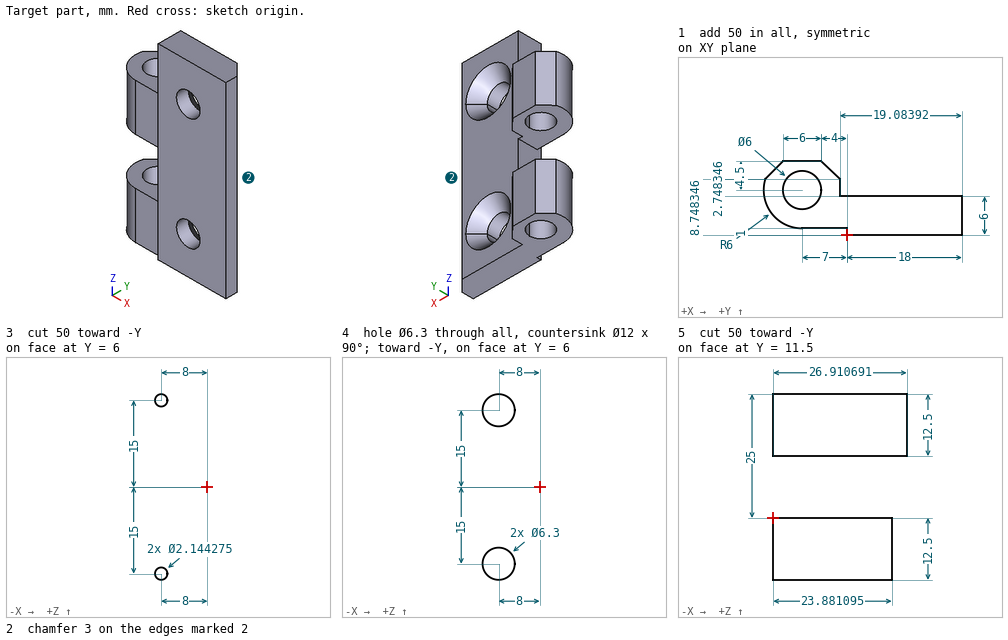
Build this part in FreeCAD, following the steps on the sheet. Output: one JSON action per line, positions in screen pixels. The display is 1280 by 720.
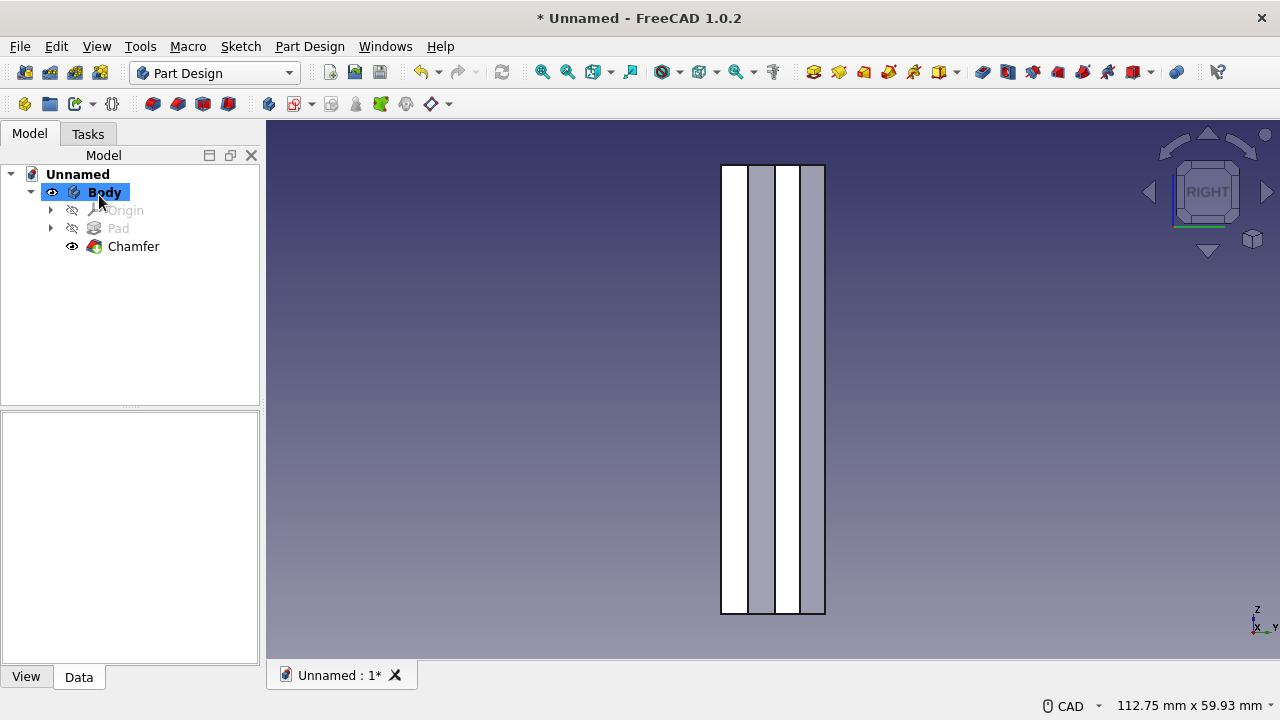
{"action": "key", "text": "4"}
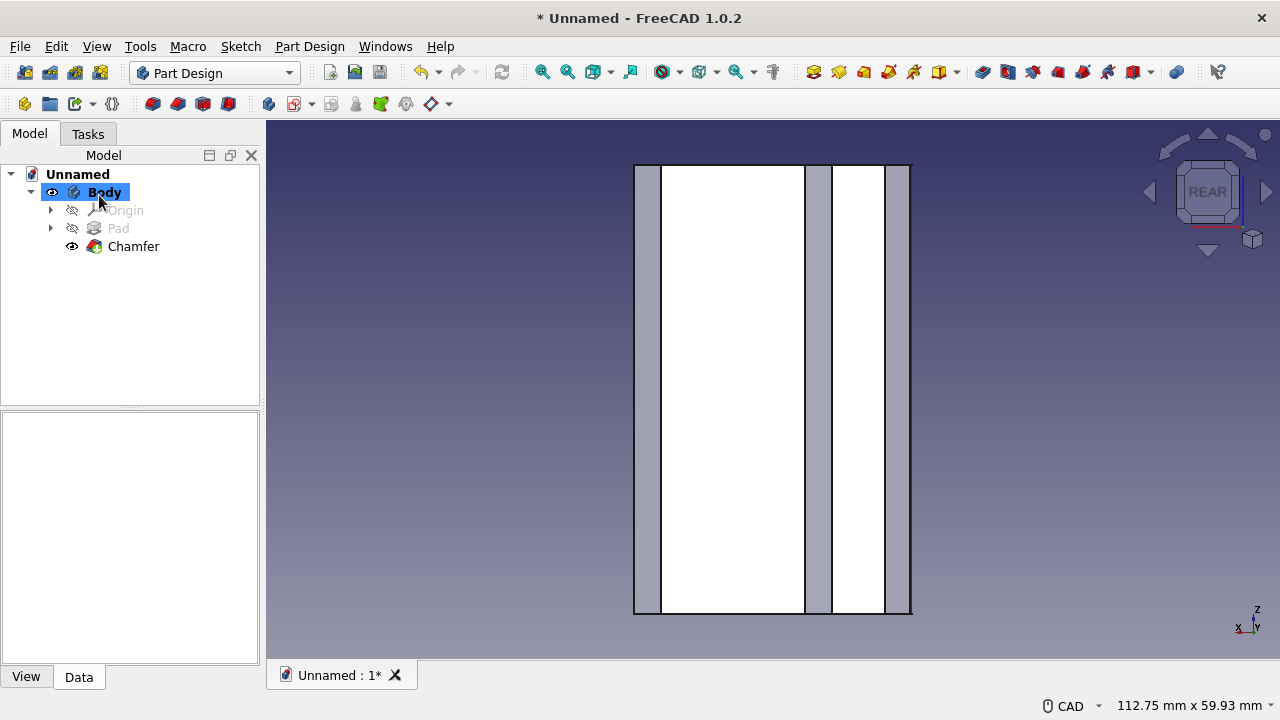
{"action": "left_click", "coordinate": [733, 260]}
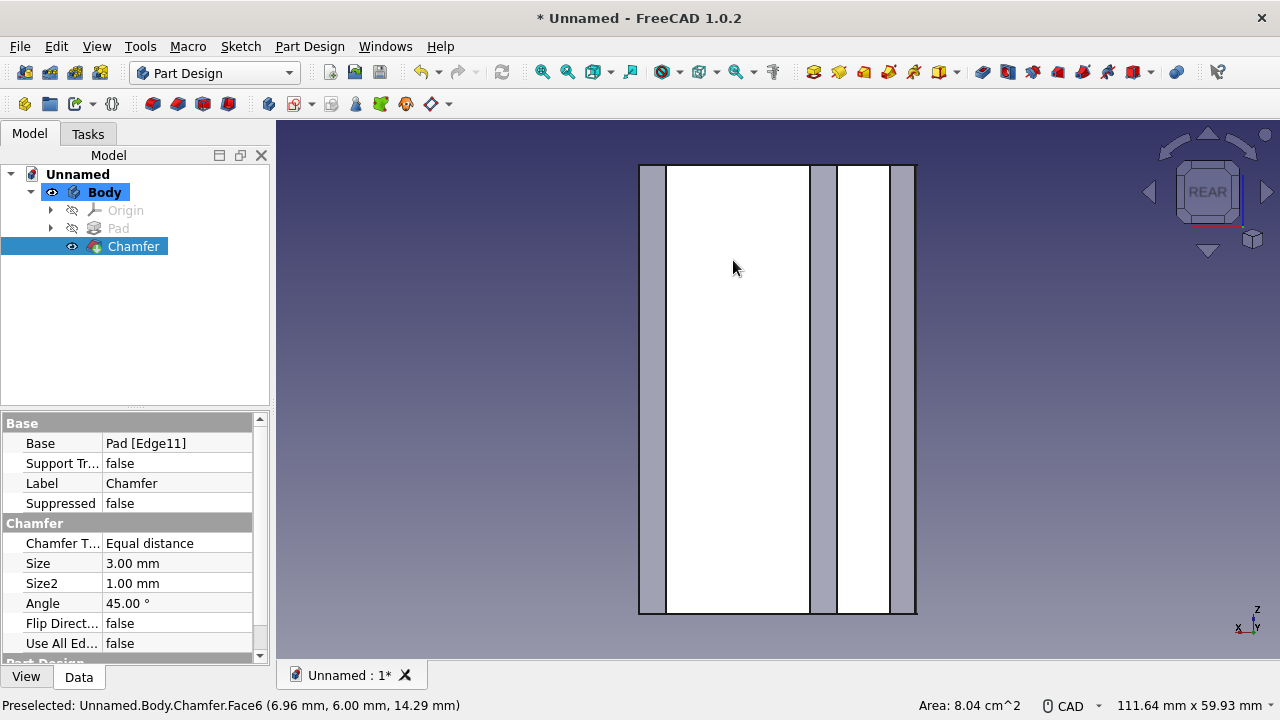
{"action": "left_click", "coordinate": [294, 104]}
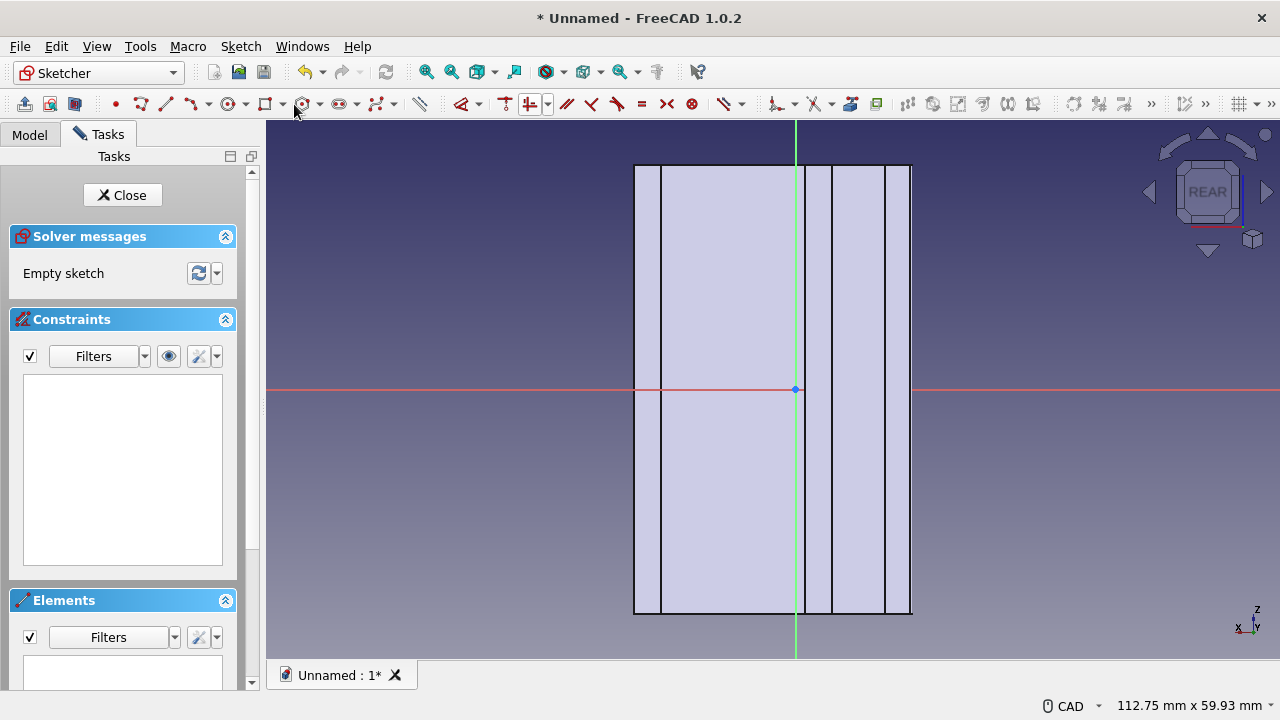
{"action": "left_click", "coordinate": [75, 104]}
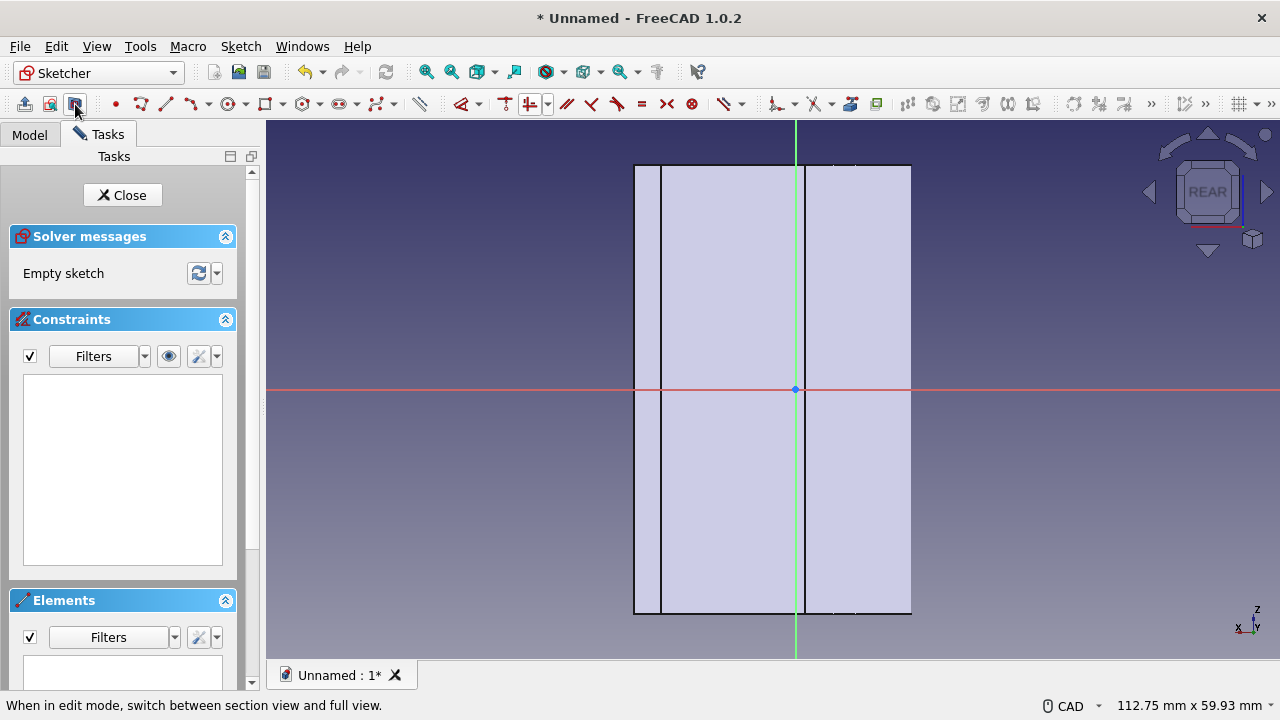
{"action": "left_click", "coordinate": [228, 104]}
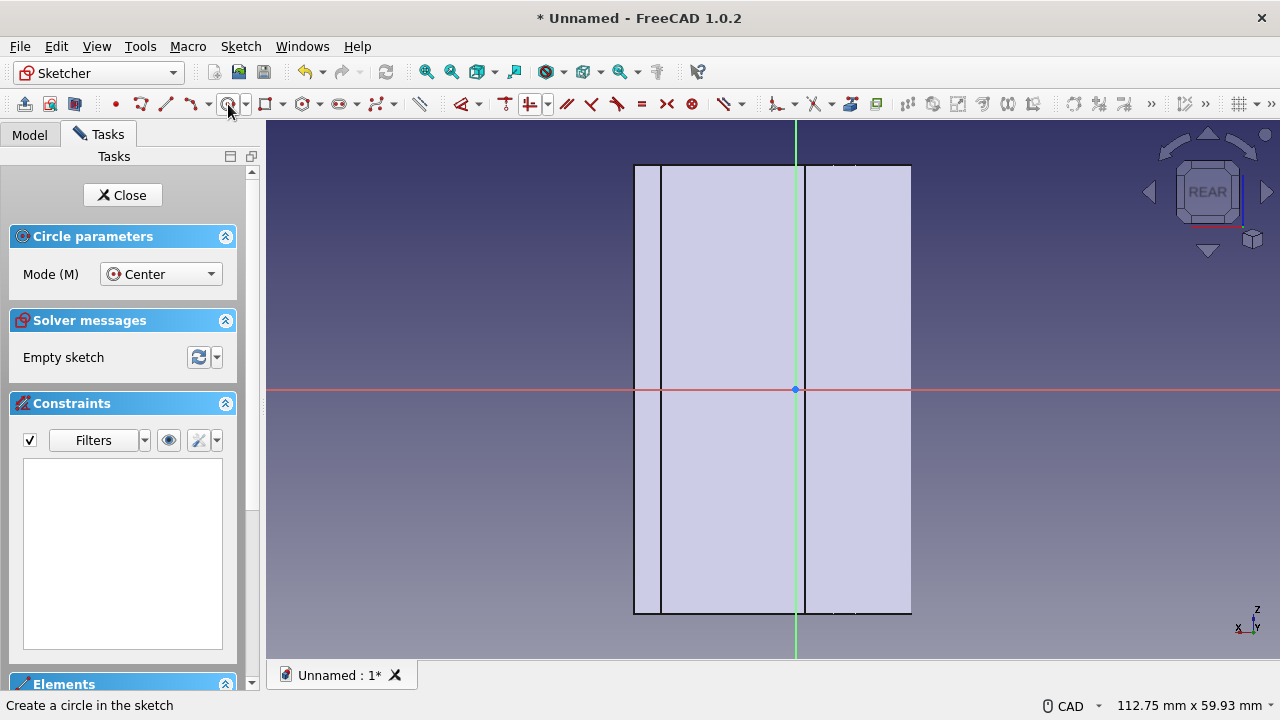
{"action": "scroll", "coordinate": [724, 524], "scroll_direction": "up", "scroll_amount": 5}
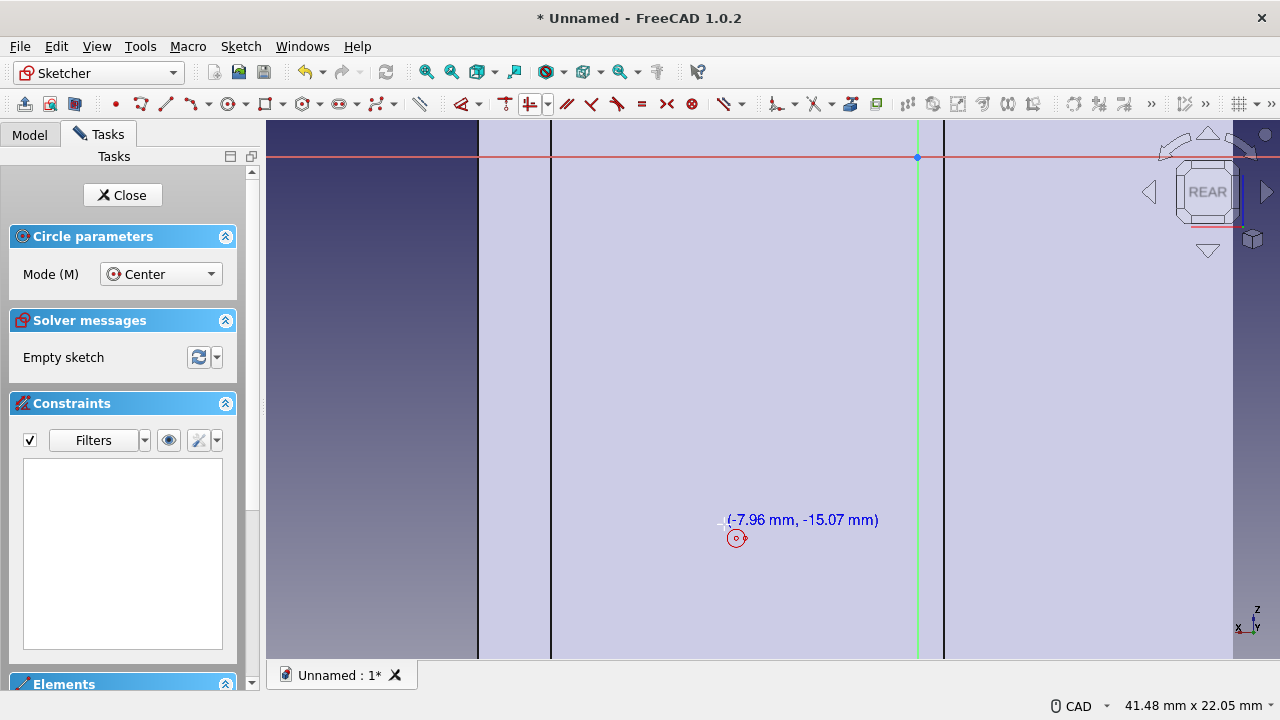
{"action": "left_click", "coordinate": [722, 524]}
{"action": "mouse_move", "coordinate": [741, 505]}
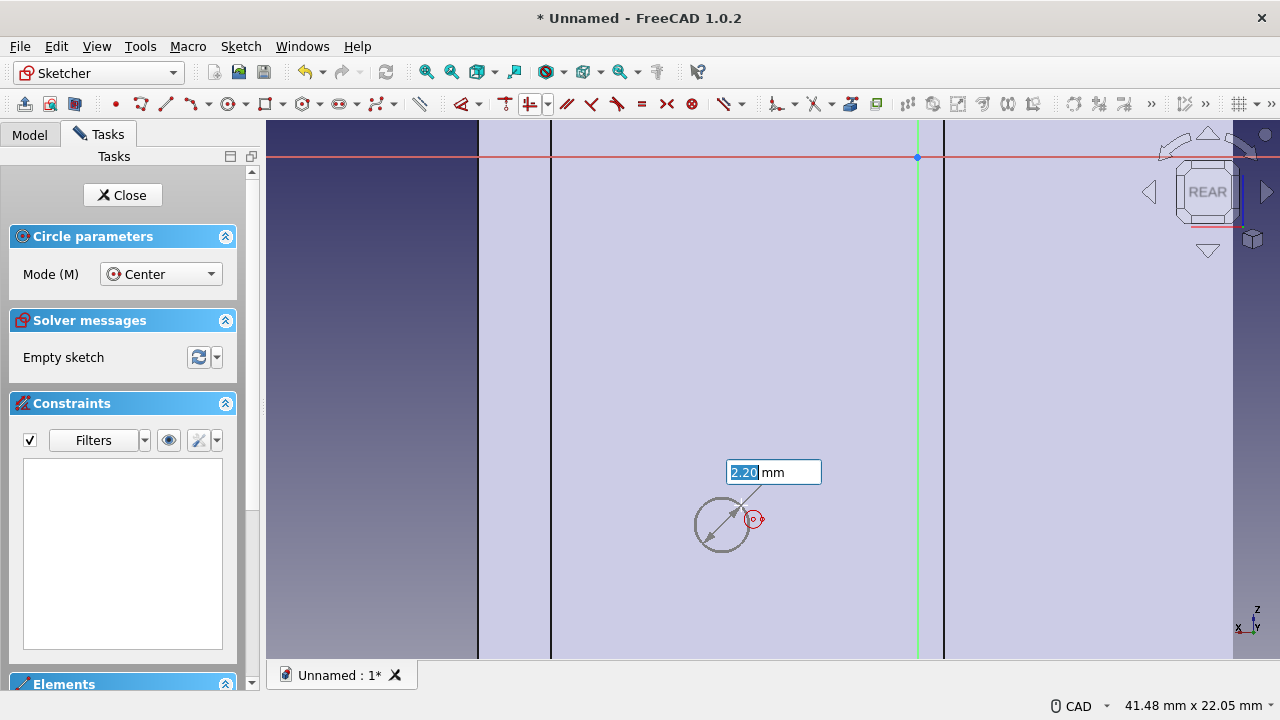
{"action": "type", "text": "2.144275"}
{"action": "key", "text": "Return"}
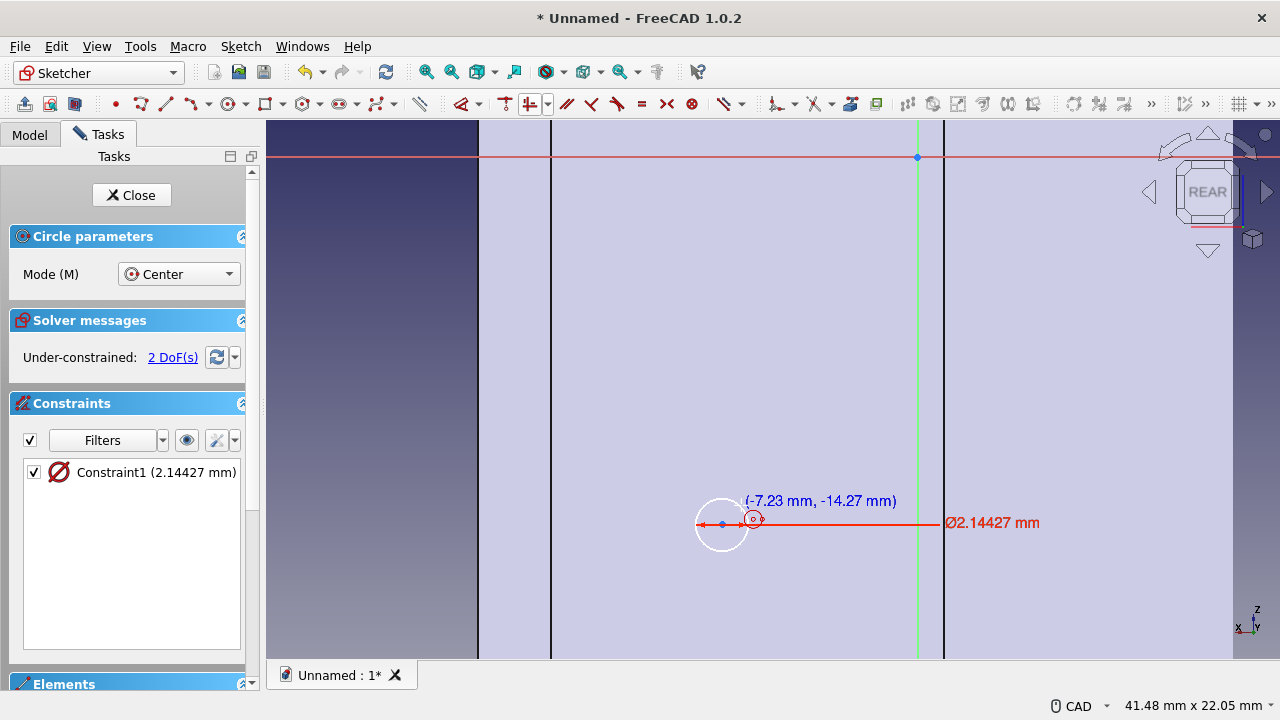
{"action": "scroll", "coordinate": [621, 579], "scroll_direction": "down", "scroll_amount": 4}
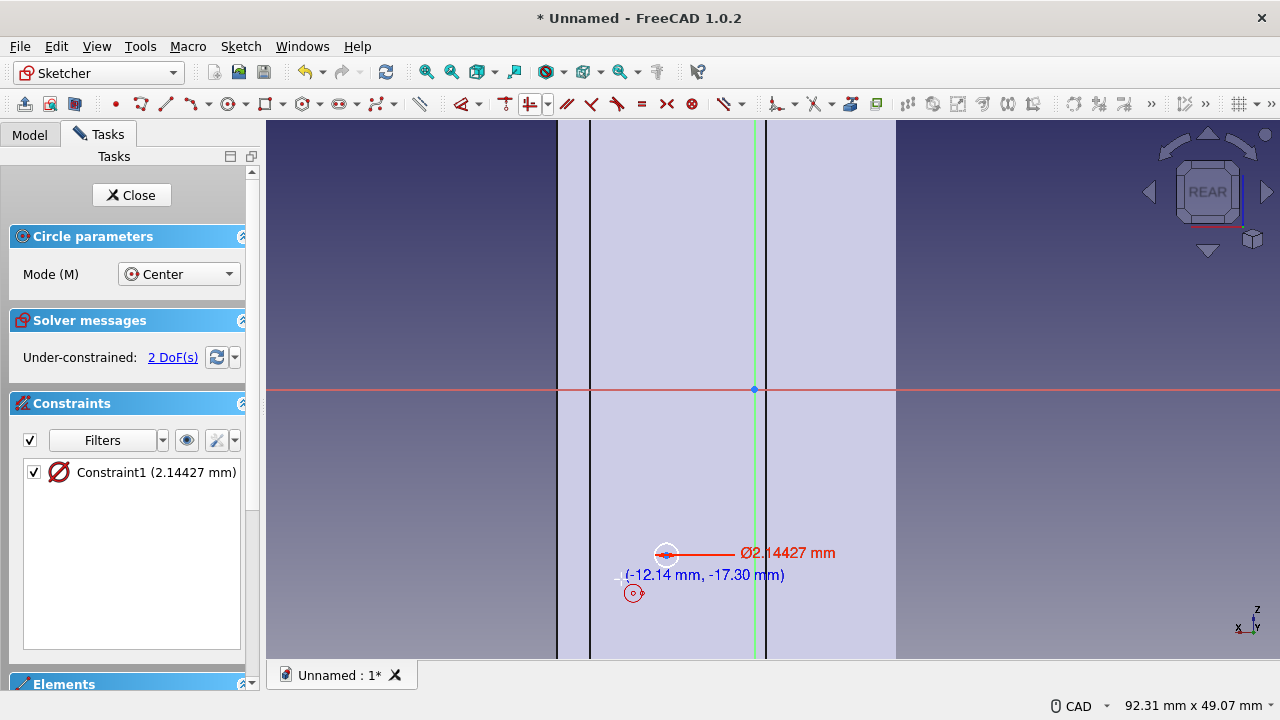
{"action": "scroll", "coordinate": [667, 225], "scroll_direction": "up", "scroll_amount": 4}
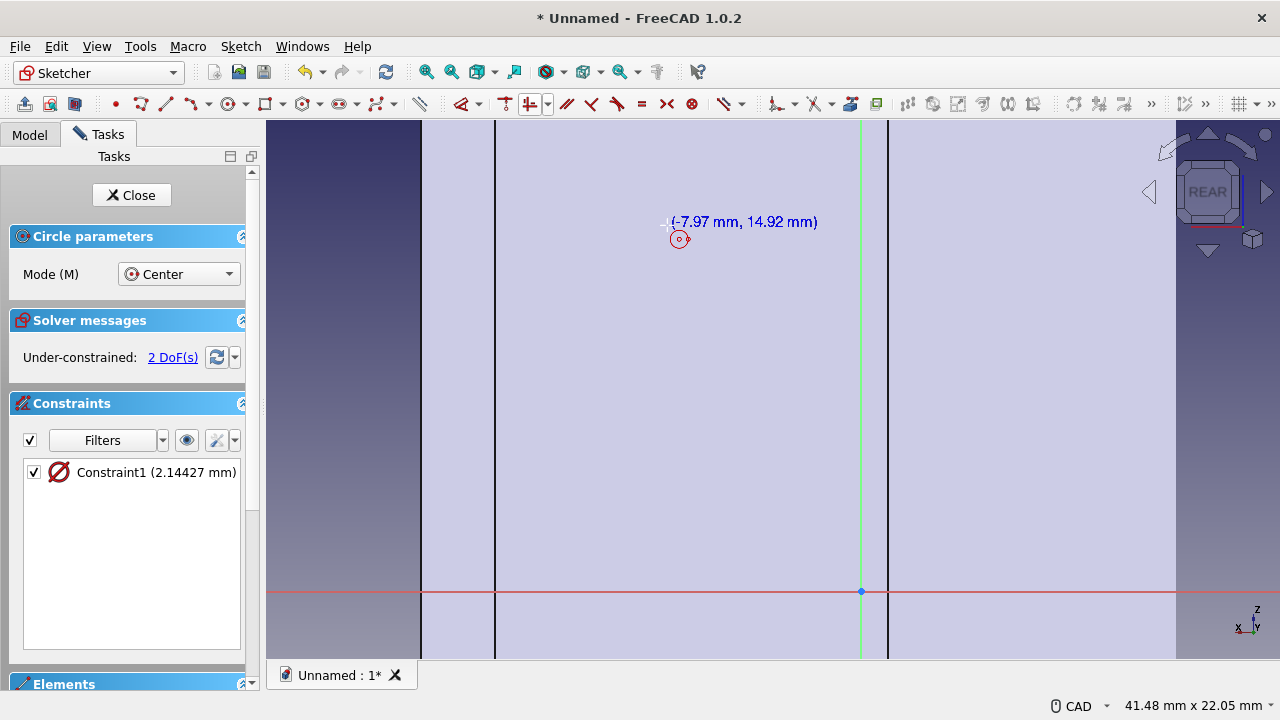
{"action": "left_click", "coordinate": [666, 225]}
{"action": "mouse_move", "coordinate": [684, 207]}